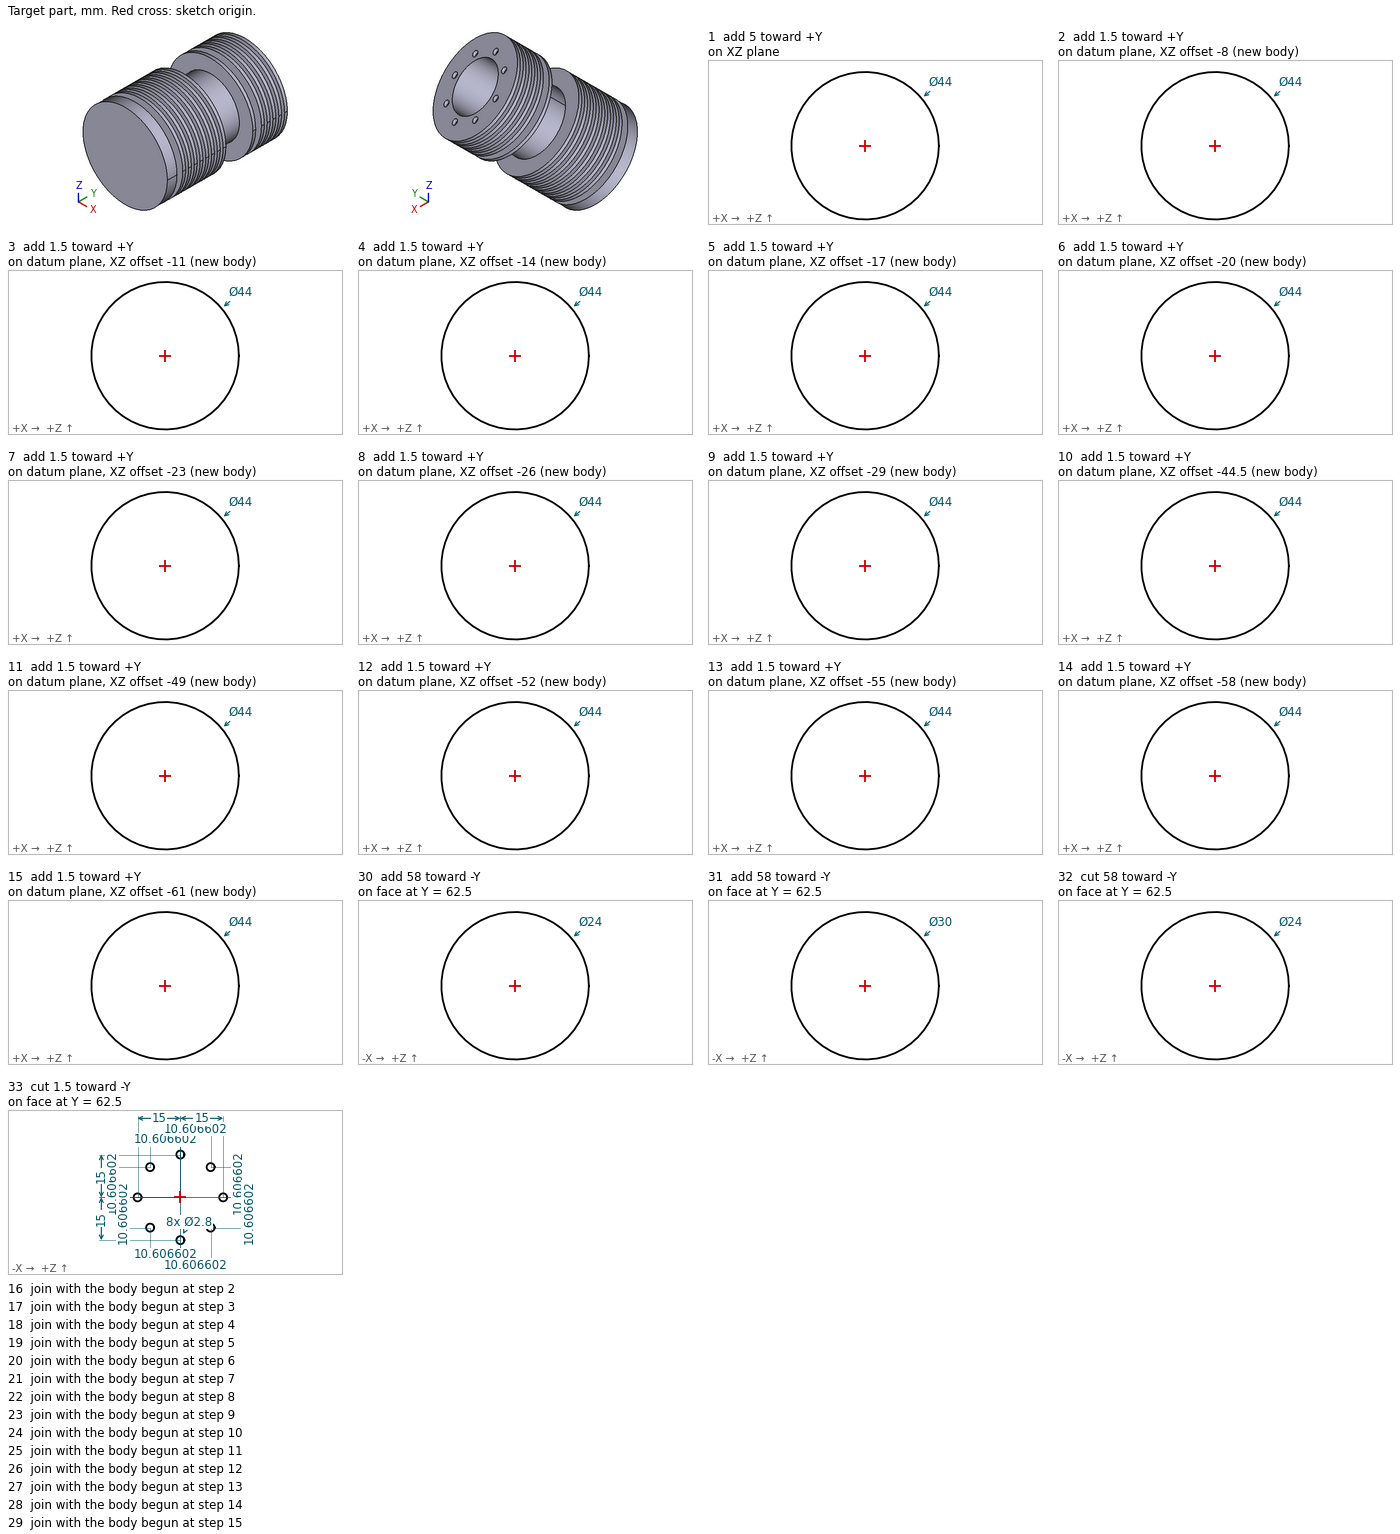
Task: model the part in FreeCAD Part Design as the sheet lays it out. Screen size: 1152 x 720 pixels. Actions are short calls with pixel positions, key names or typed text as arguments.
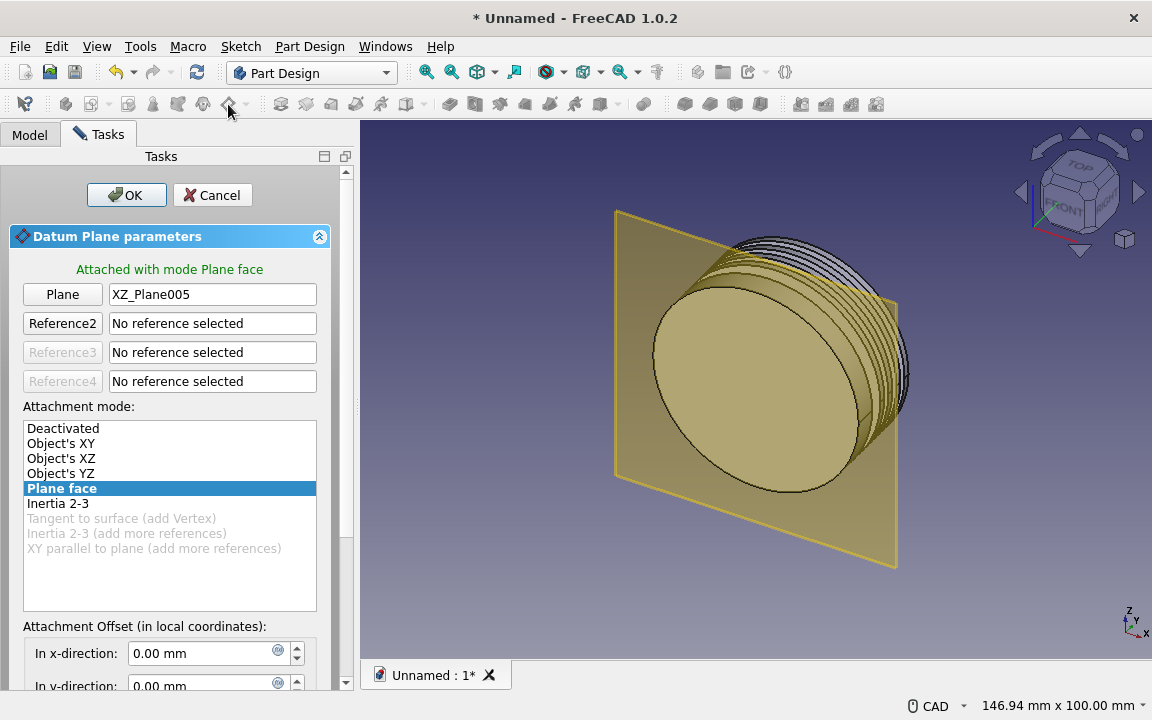
scroll(346, 428, down, 2)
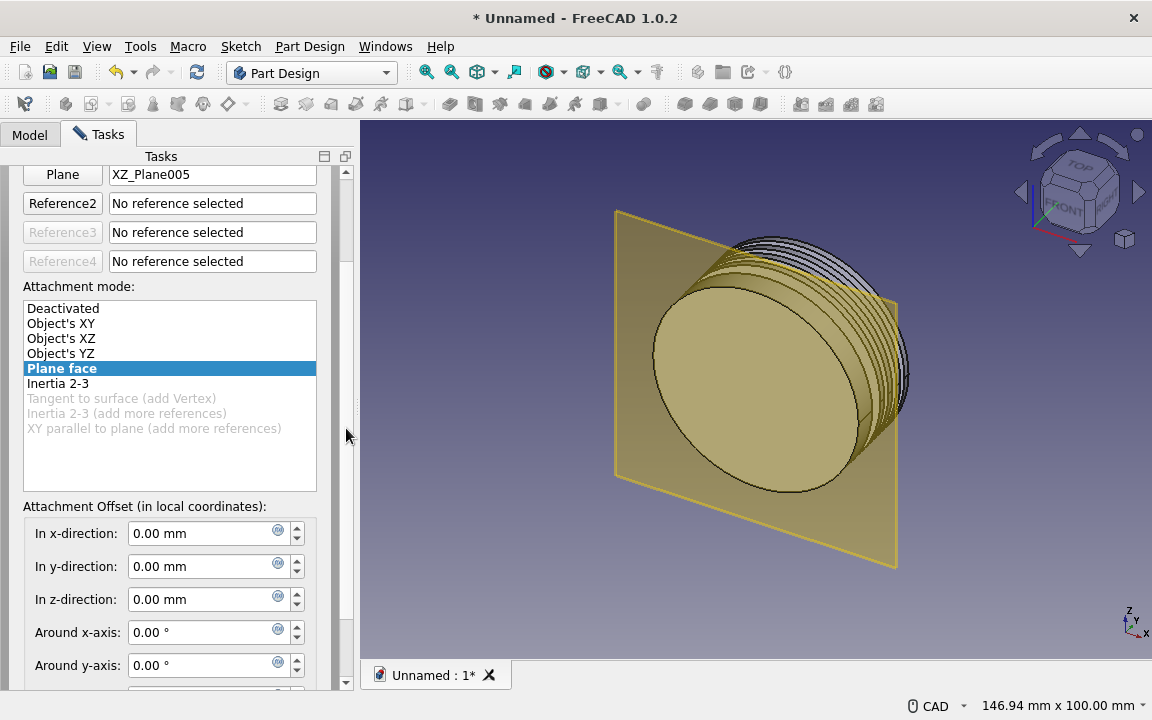
triple_click(210, 600)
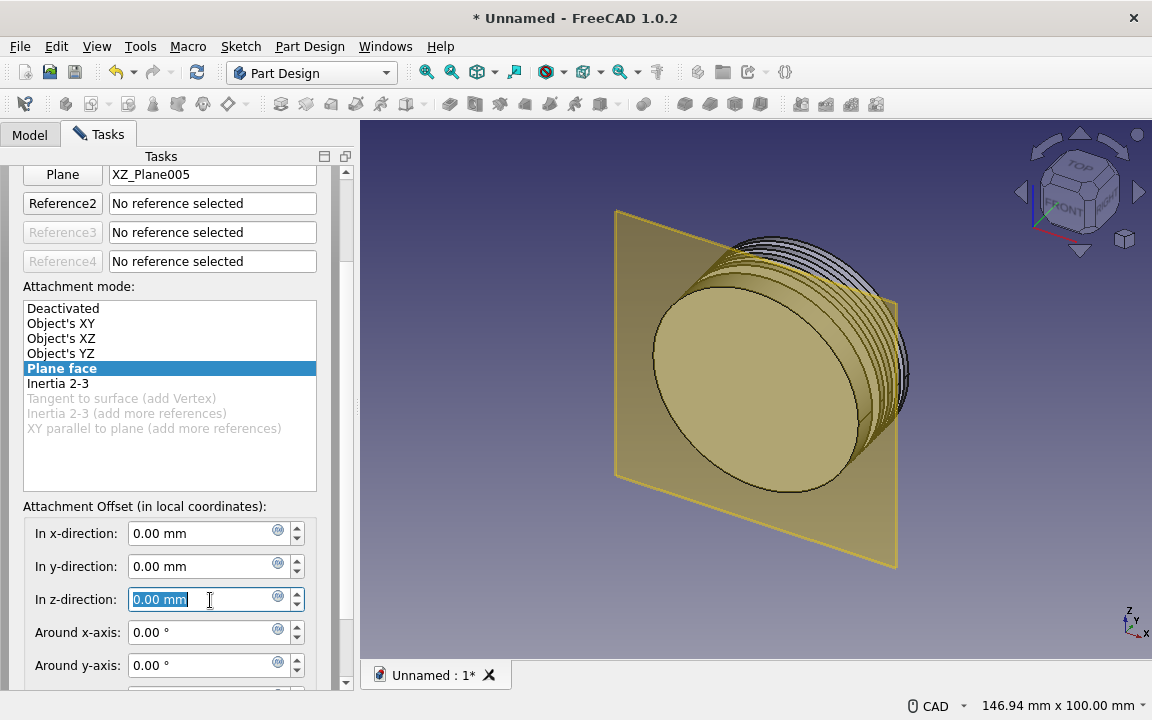
text(-20)
key(Tab)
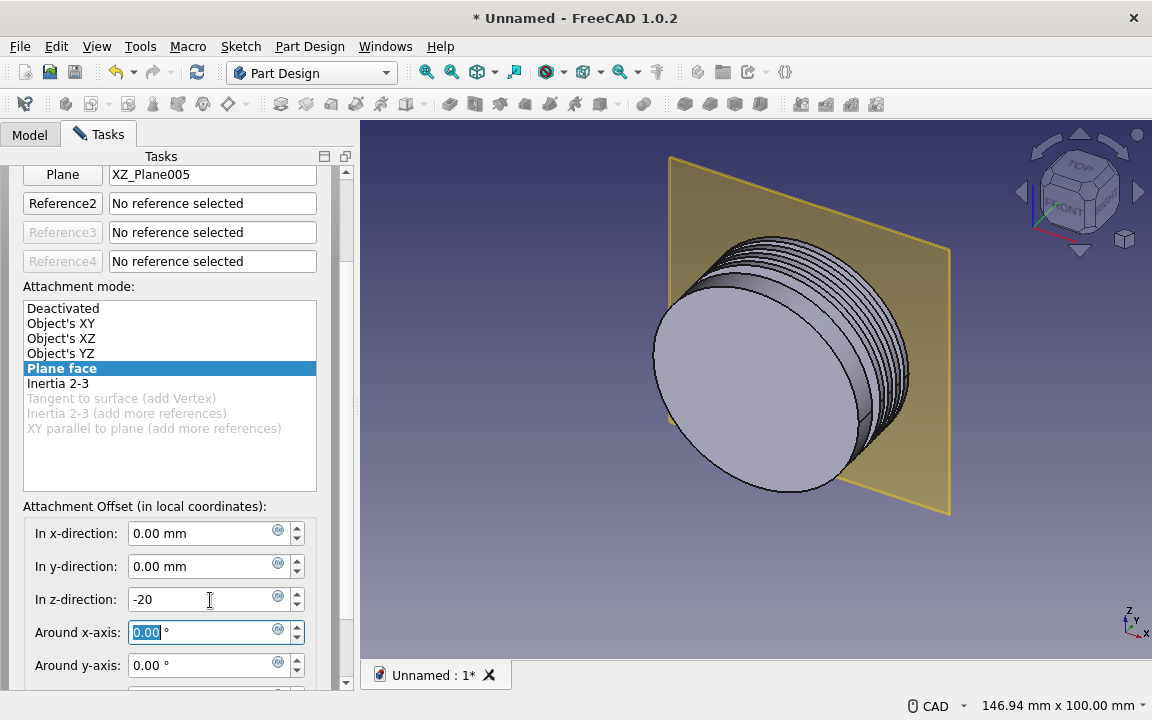
scroll(346, 428, up, 3)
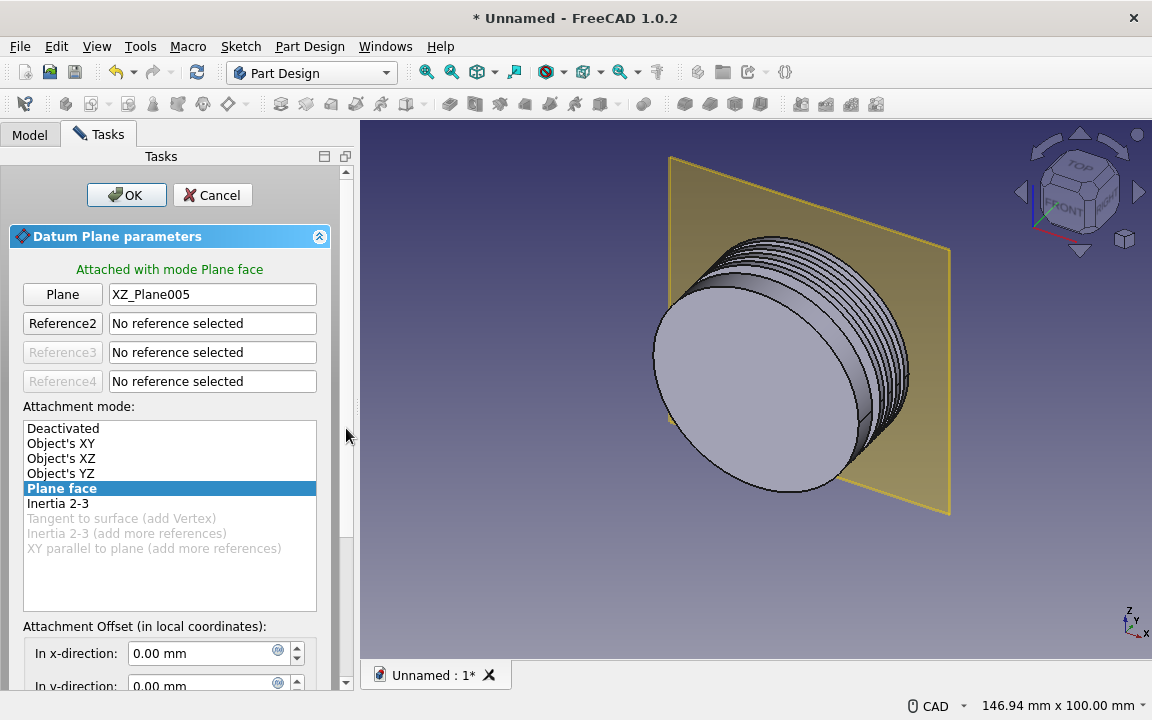
click(127, 195)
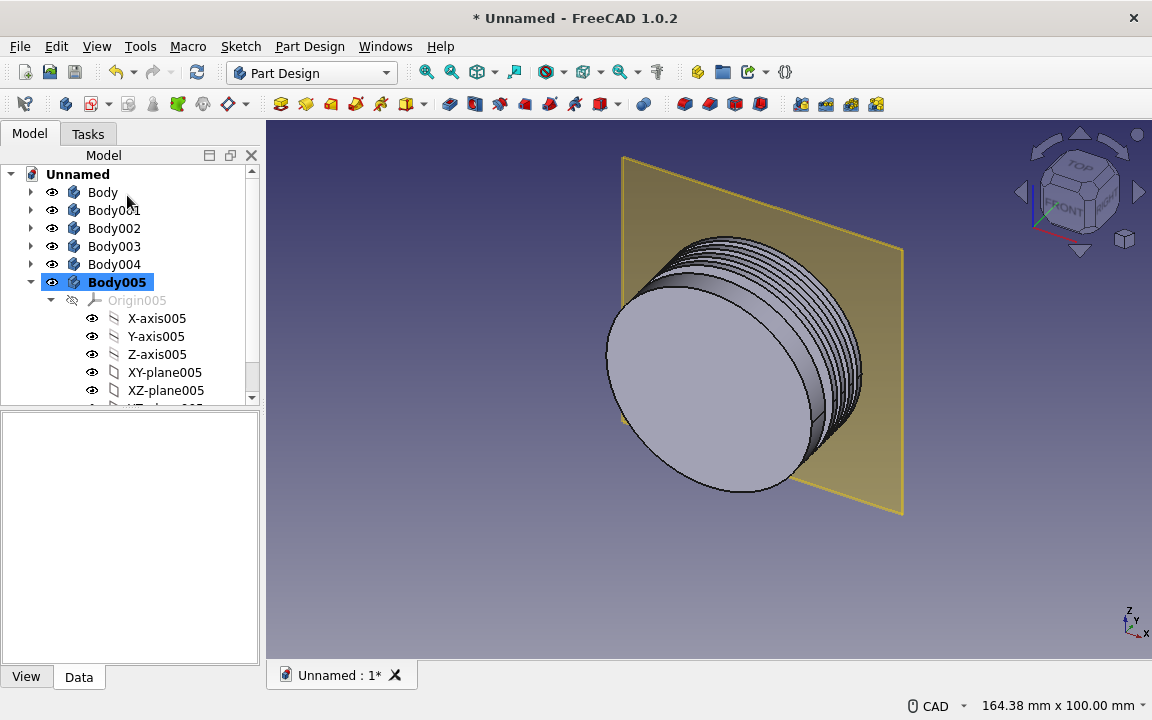
scroll(101, 278, down, 3)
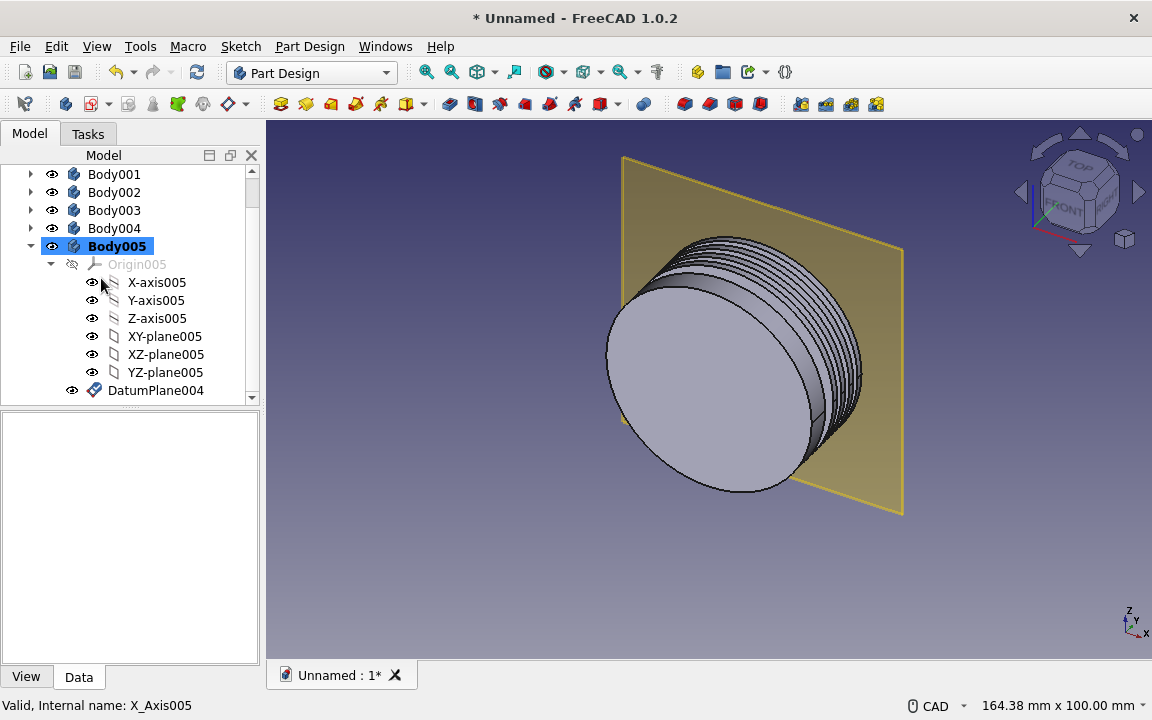
click(117, 390)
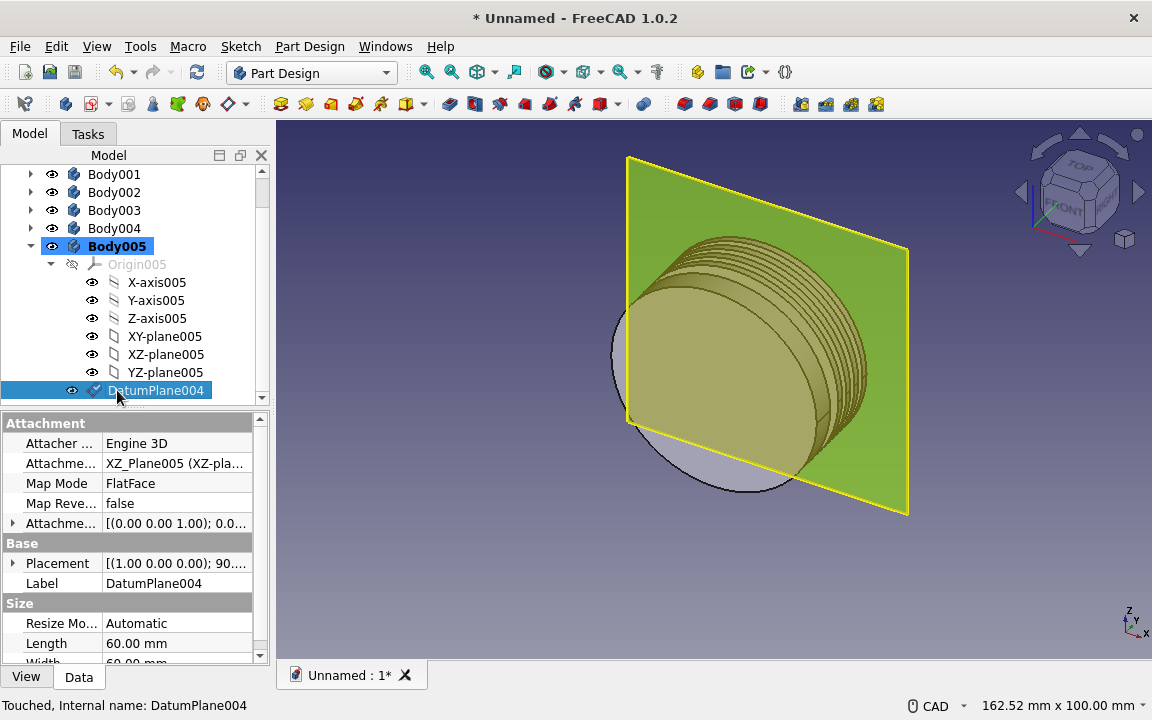
click(90, 104)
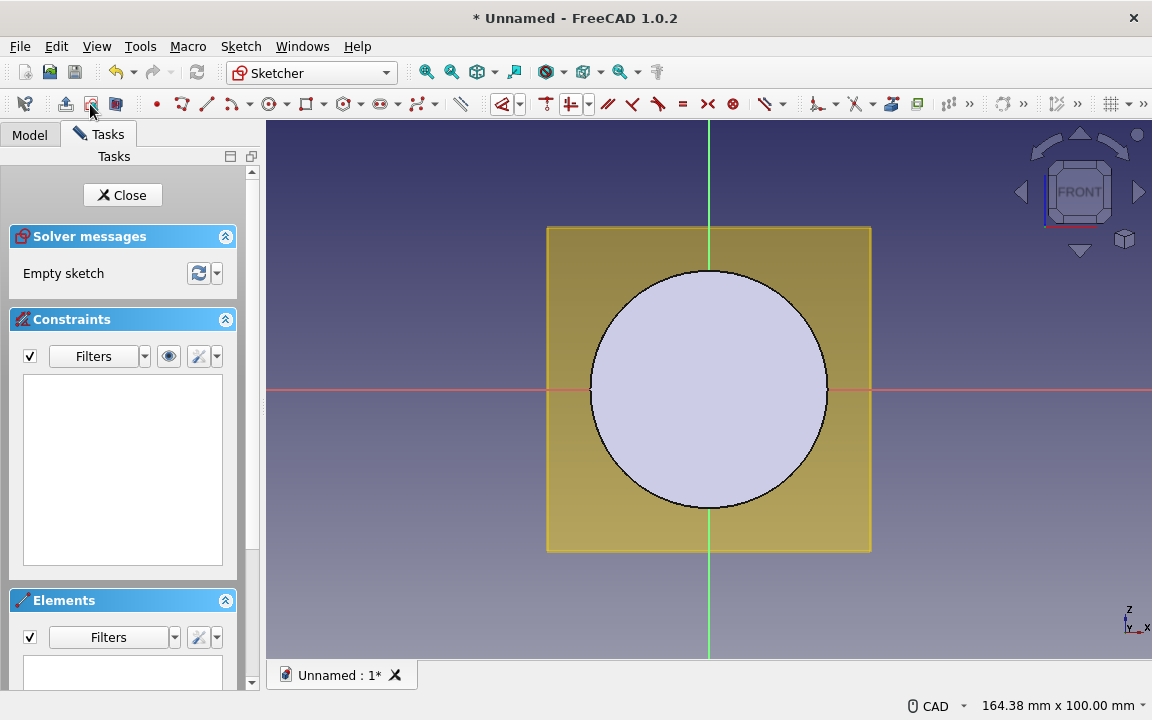
scroll(848, 390, up, 2)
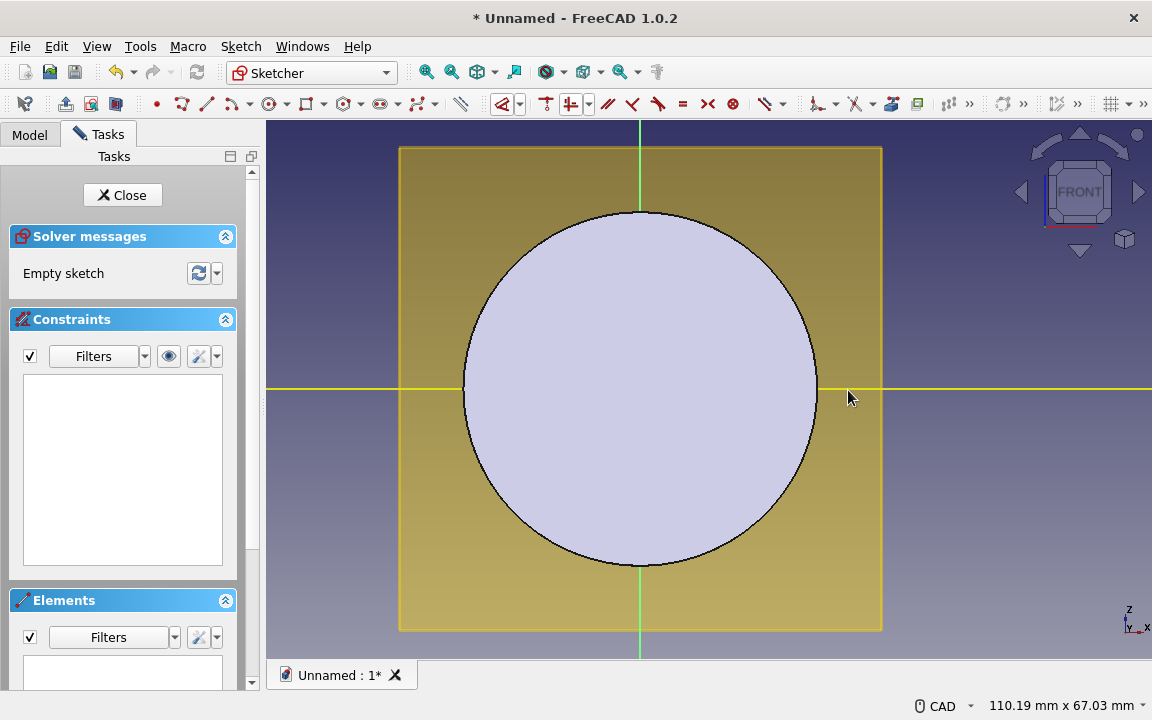
key(g)
key(c)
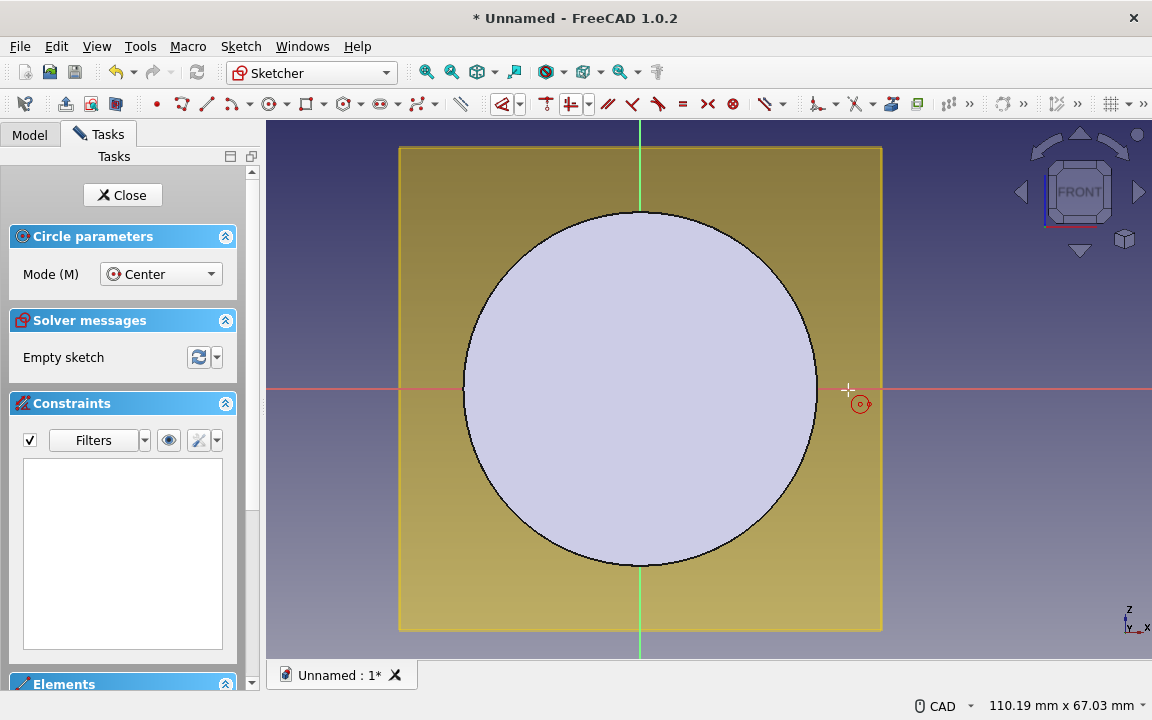
click(640, 389)
click(765, 264)
key(Escape)